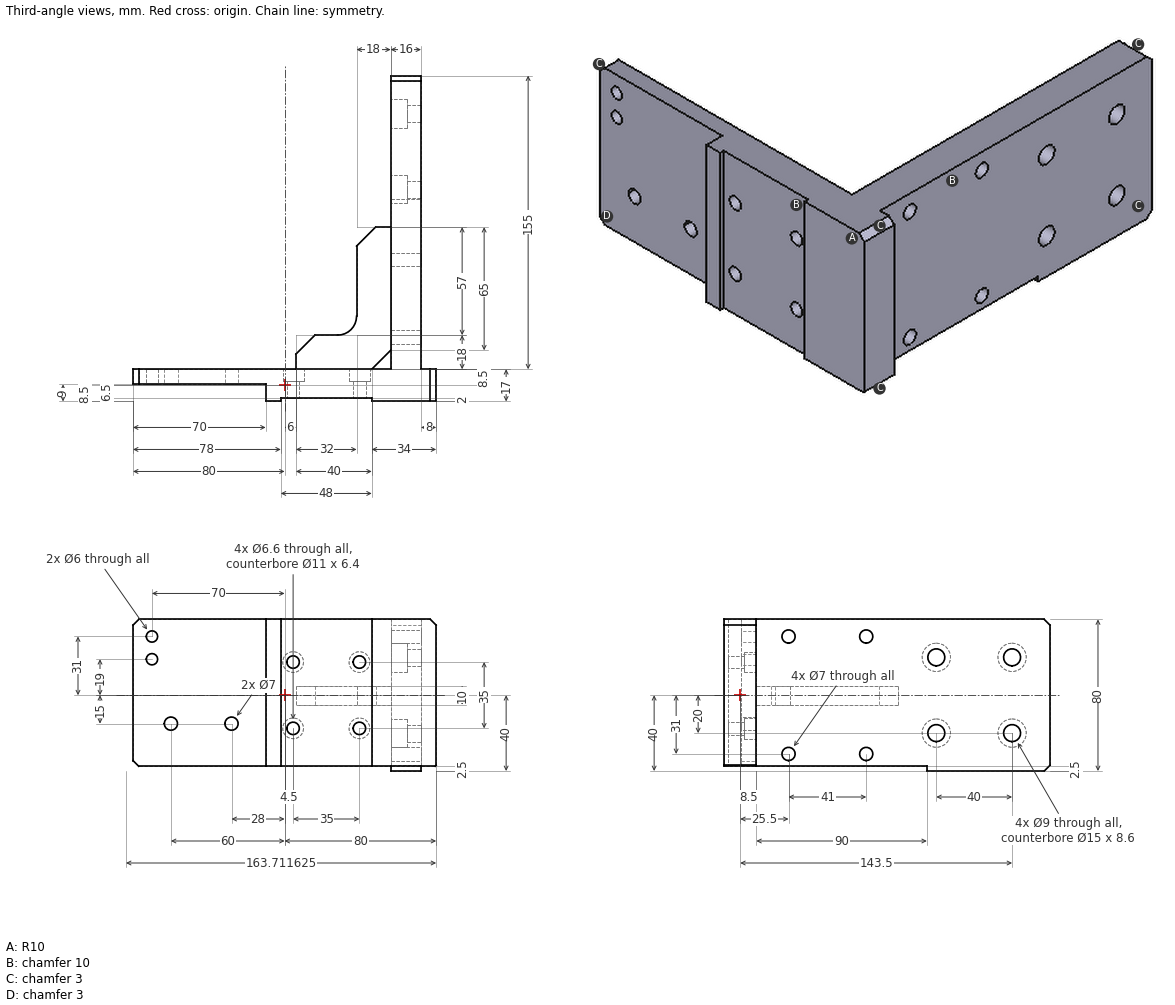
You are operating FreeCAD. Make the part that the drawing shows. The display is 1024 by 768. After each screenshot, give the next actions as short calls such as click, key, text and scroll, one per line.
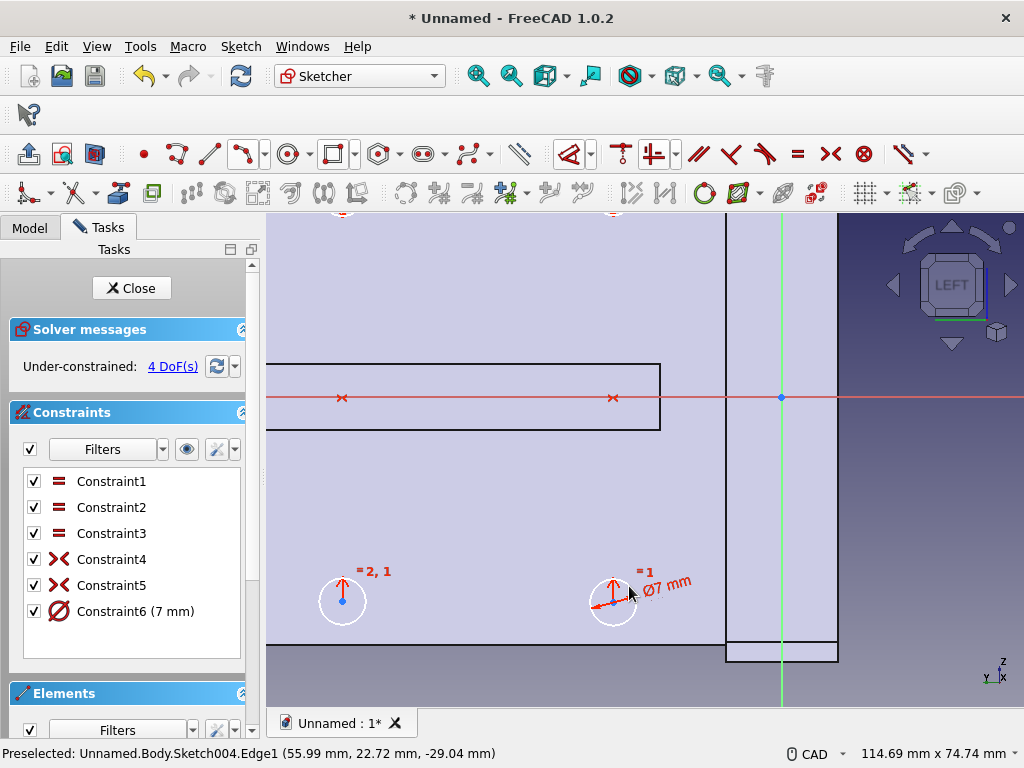
click(613, 602)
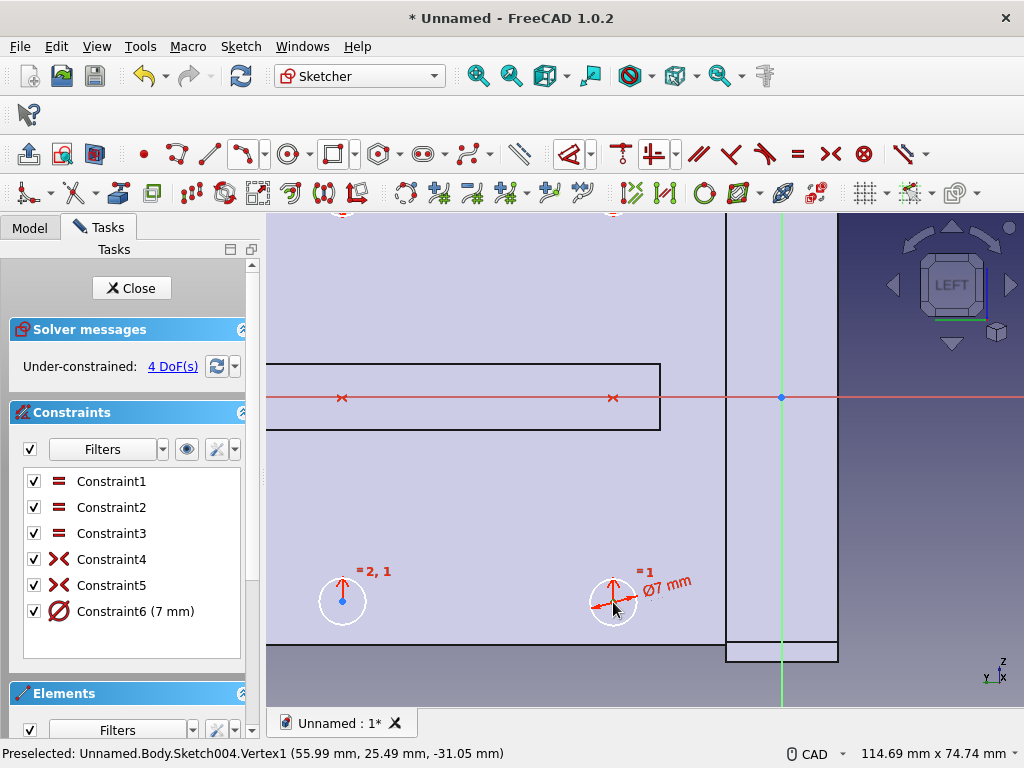
key(i)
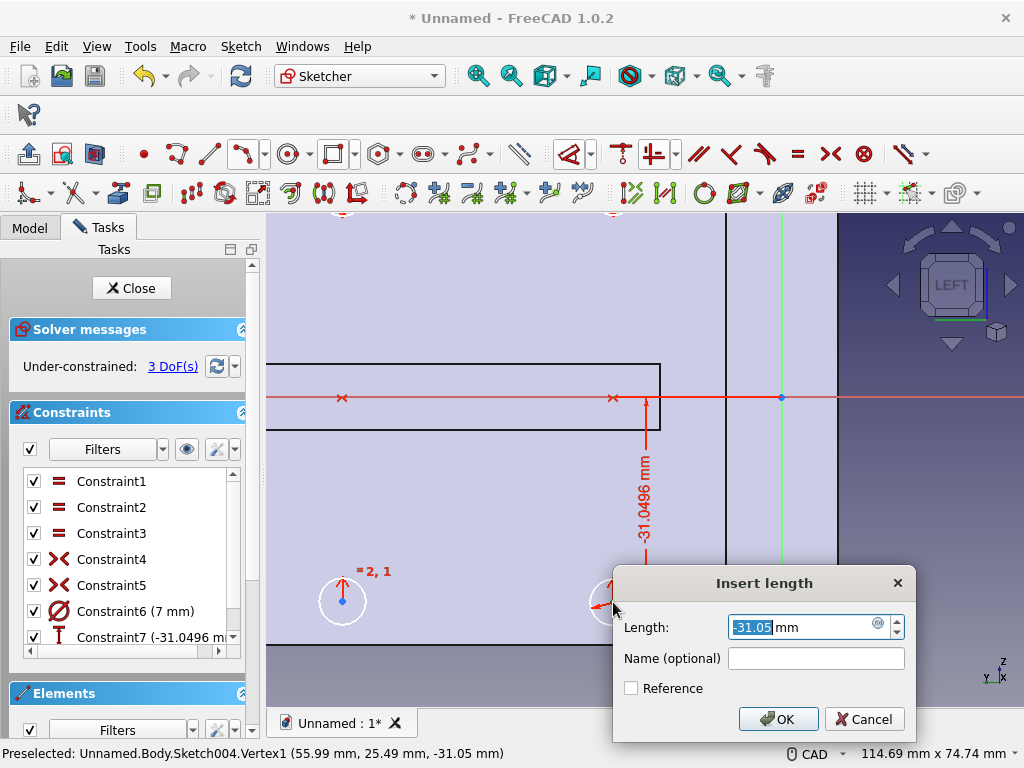
text(-31)
key(Return)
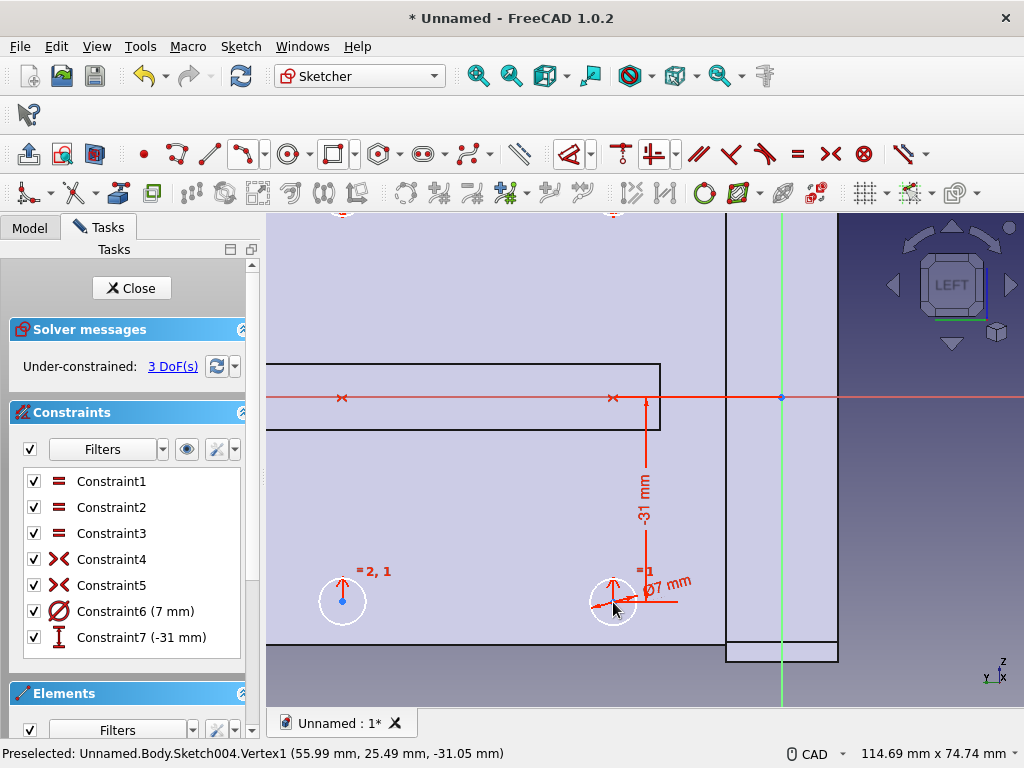
click(343, 602)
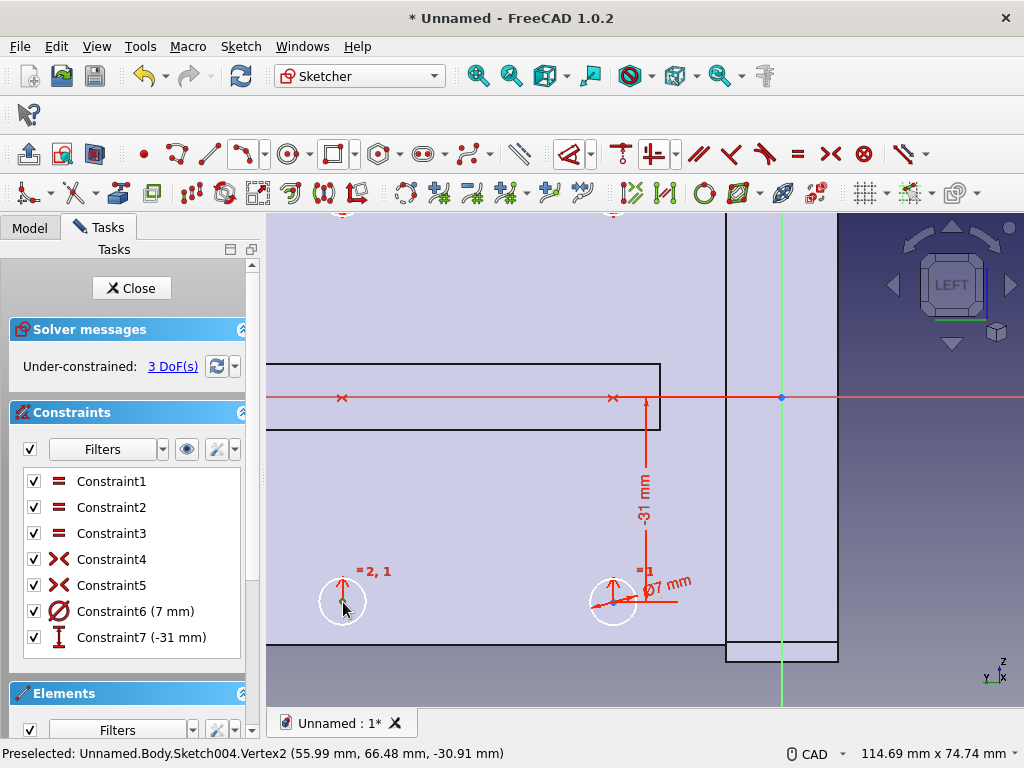
key(i)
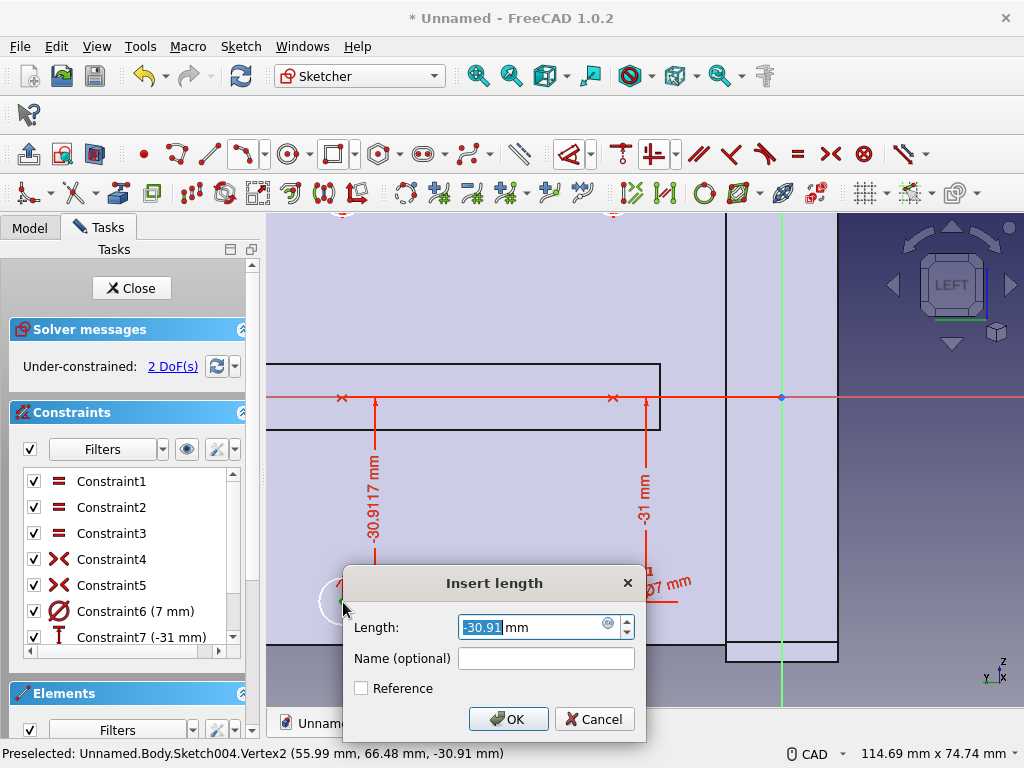
text(-31)
key(Return)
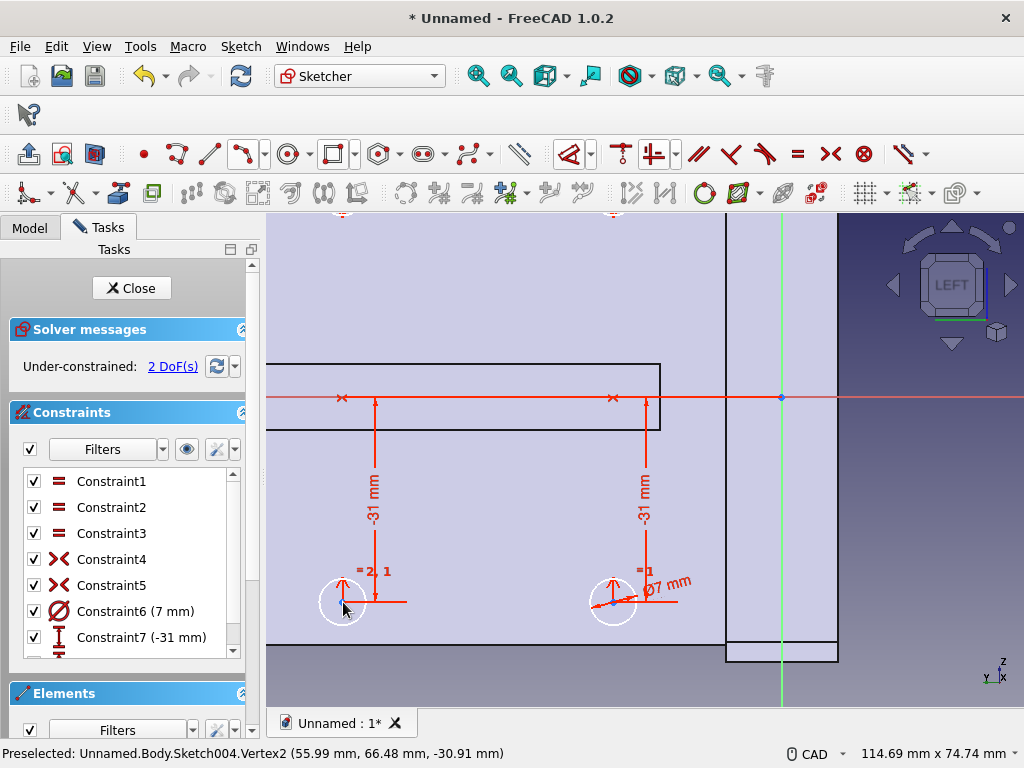
click(613, 602)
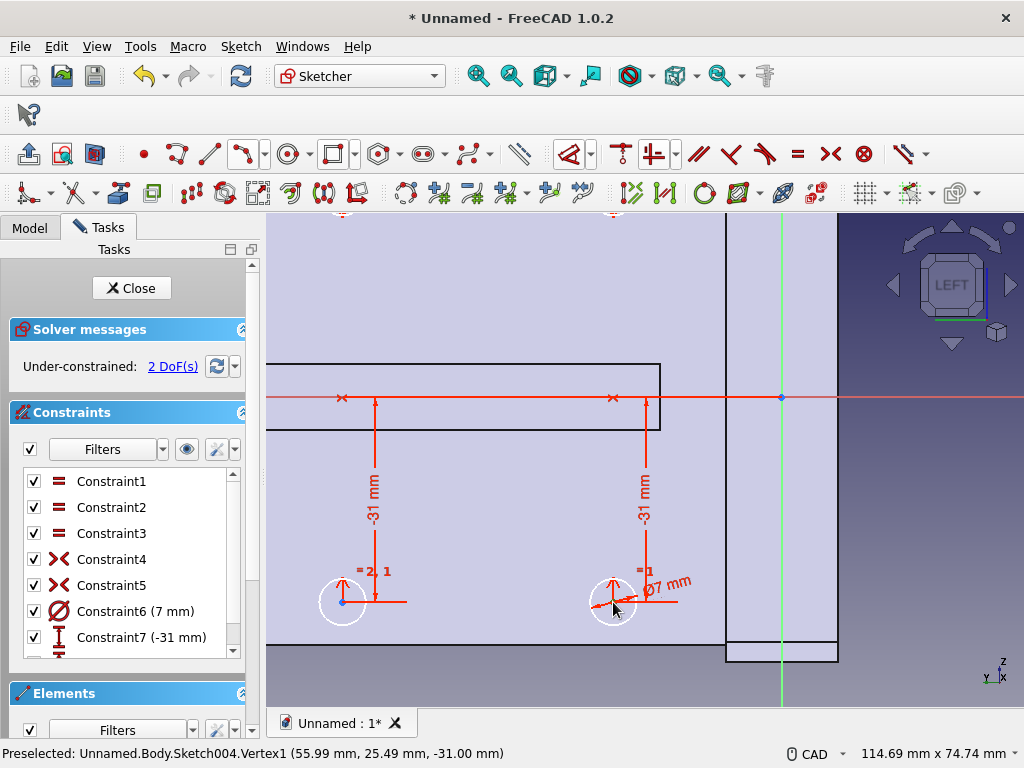
click(343, 602)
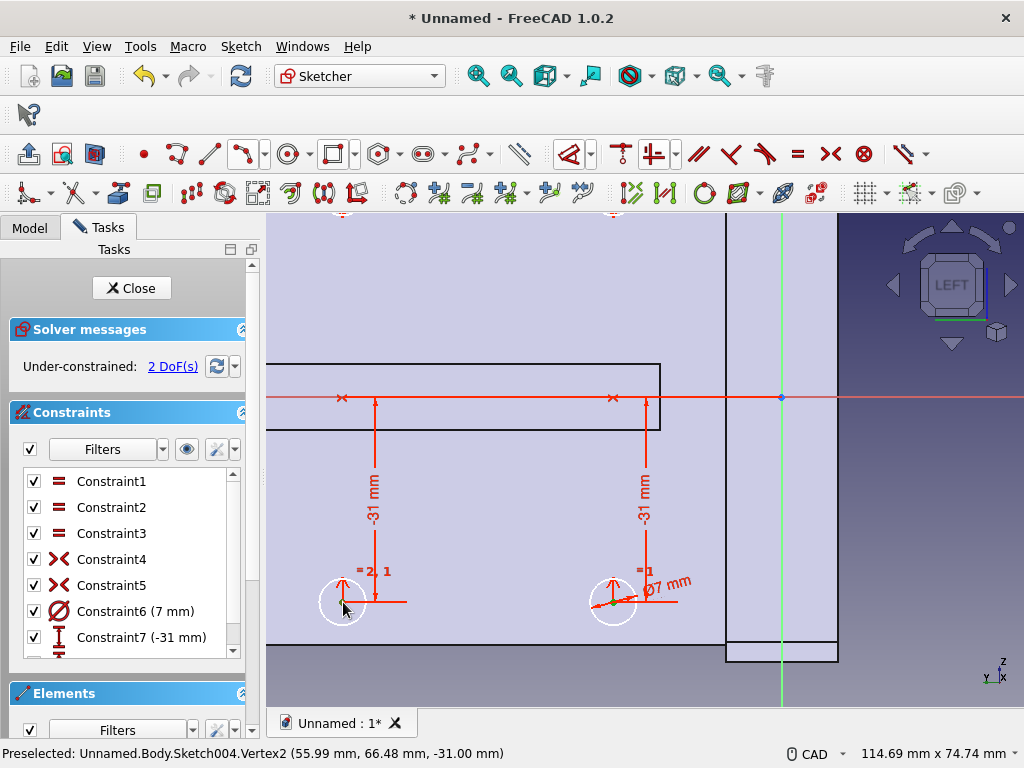
key(l)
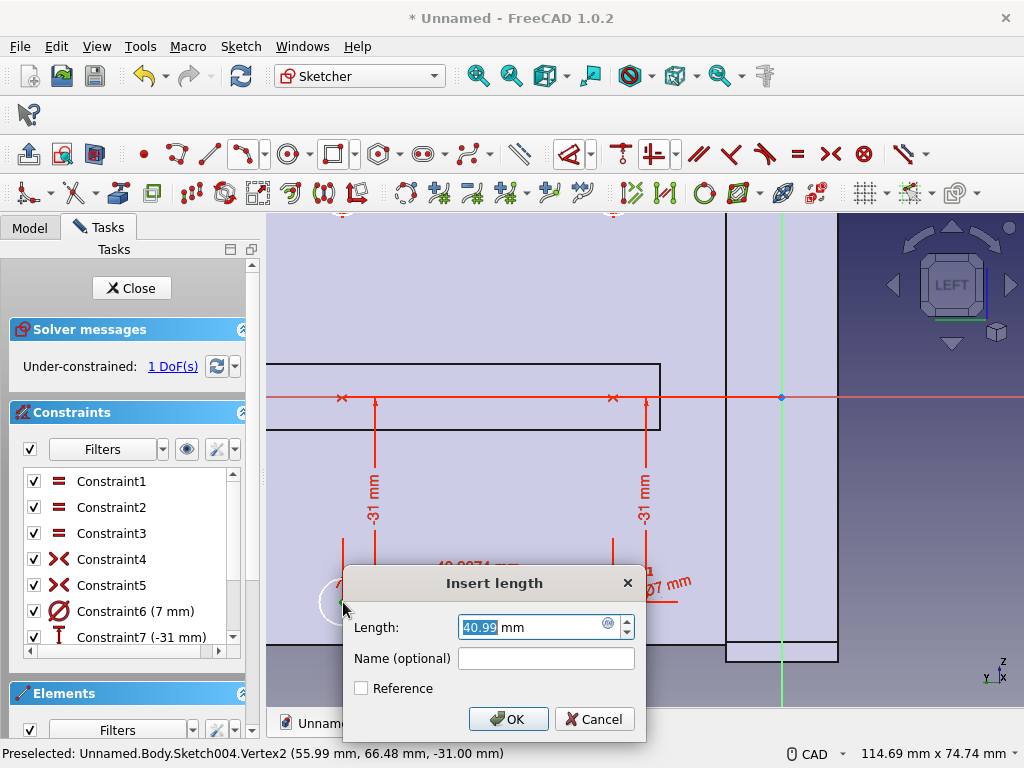
text(41)
key(Return)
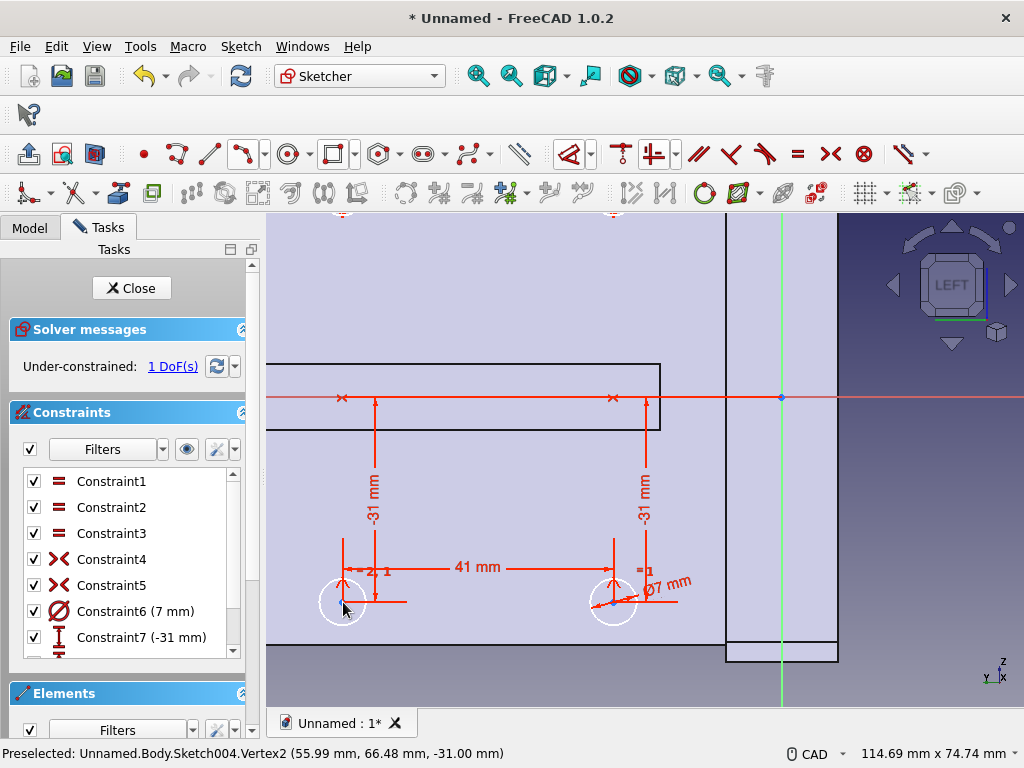
click(614, 602)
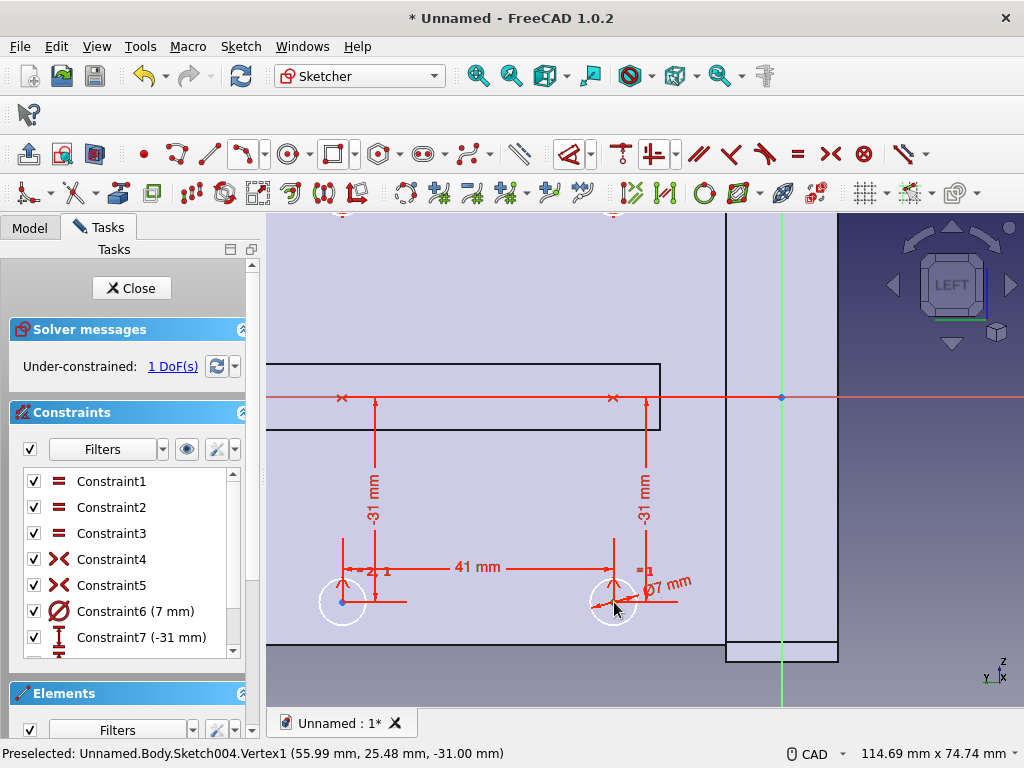
key(l)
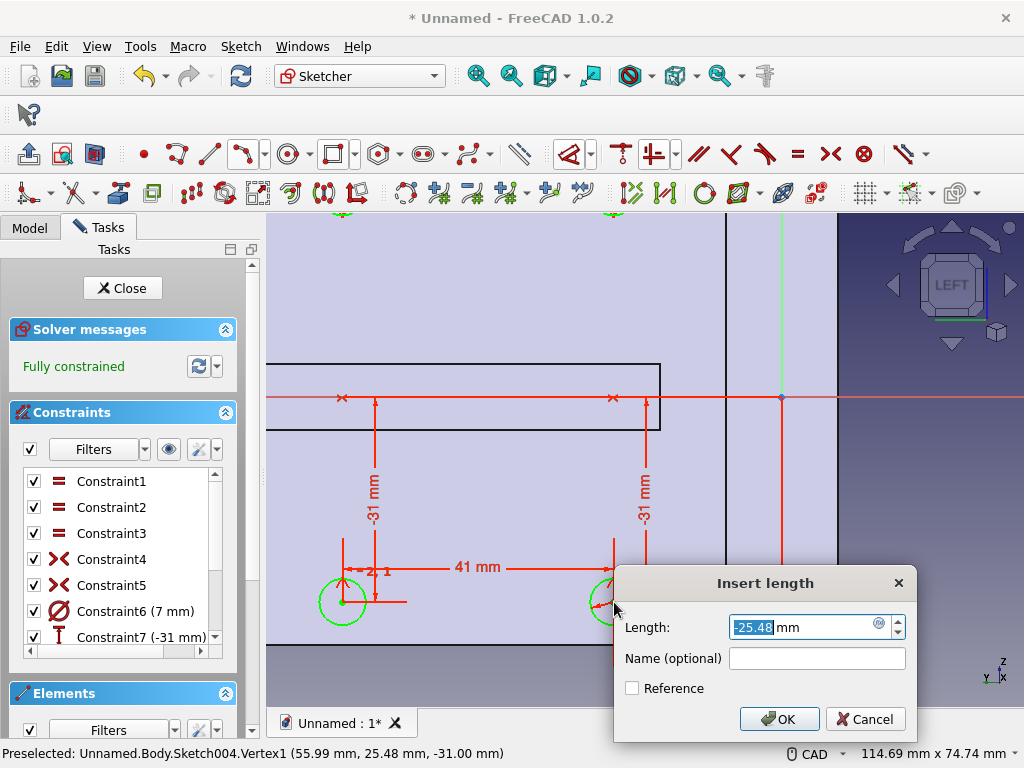
text(-25.5)
key(Return)